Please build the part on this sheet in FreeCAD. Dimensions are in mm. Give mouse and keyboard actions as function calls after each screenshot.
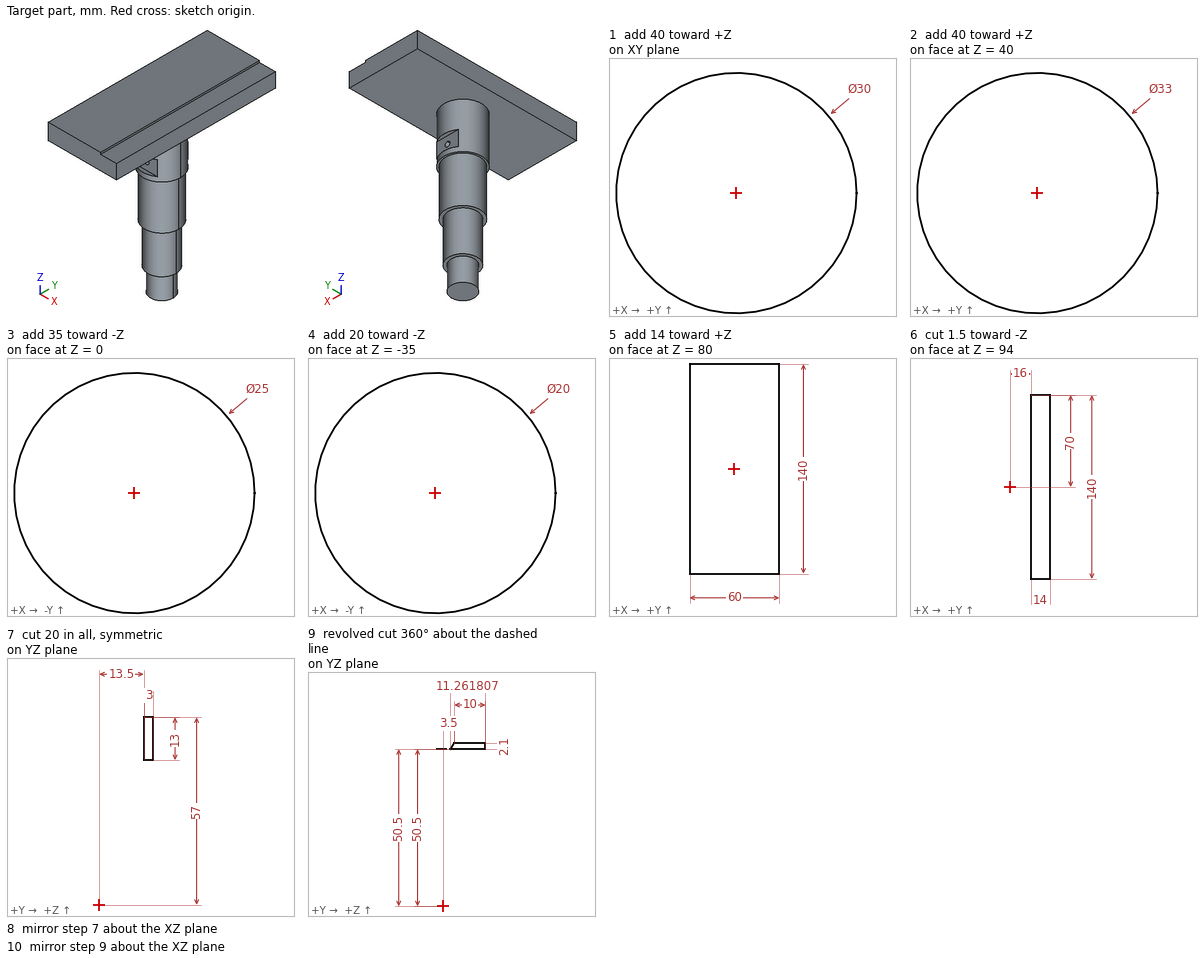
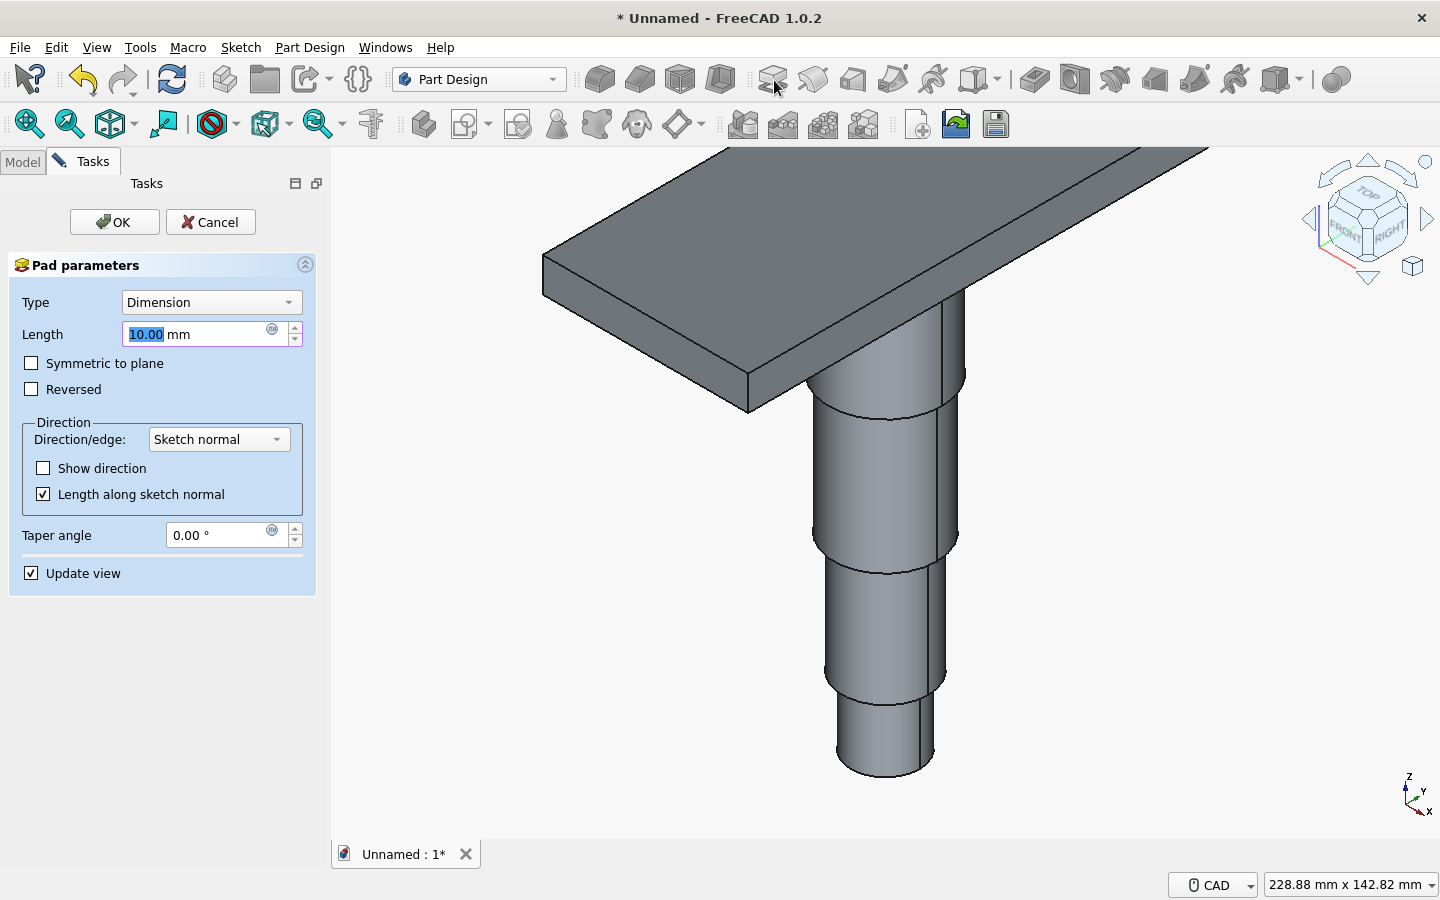
text(14)
key(Tab)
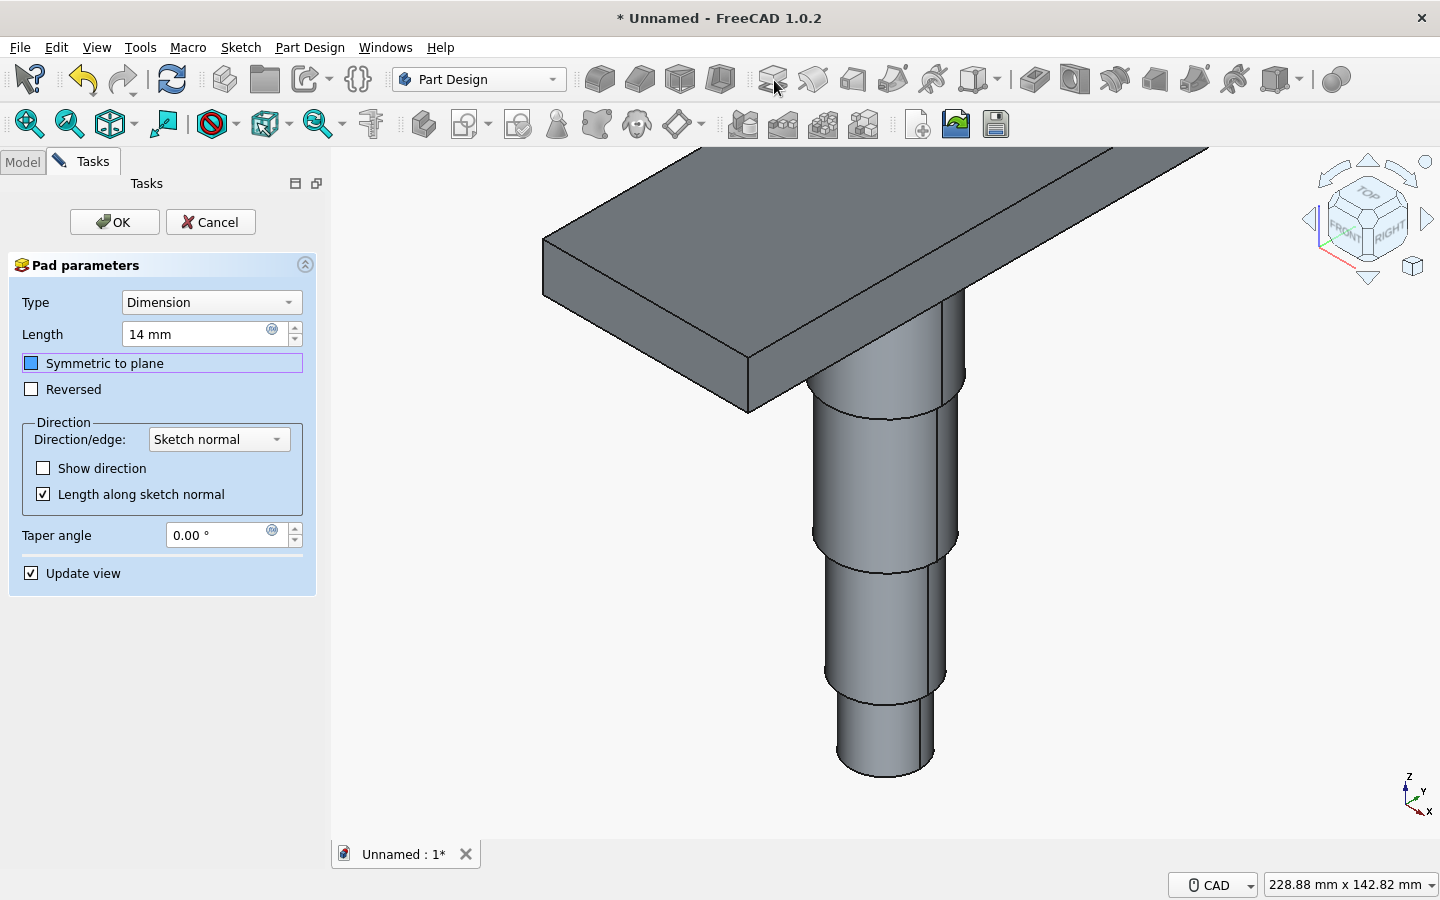
click(115, 222)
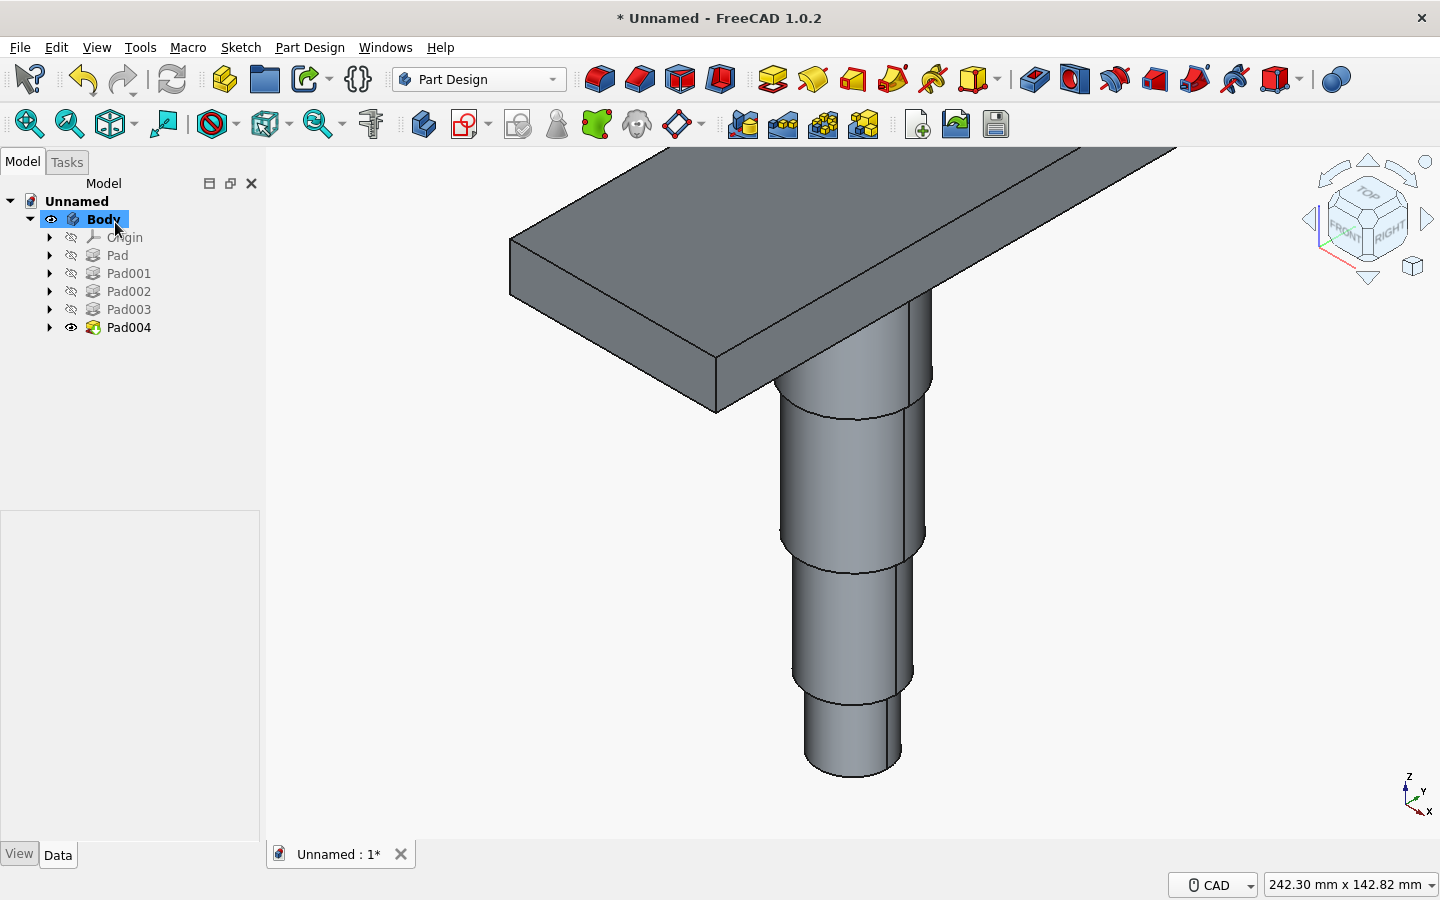
click(30, 124)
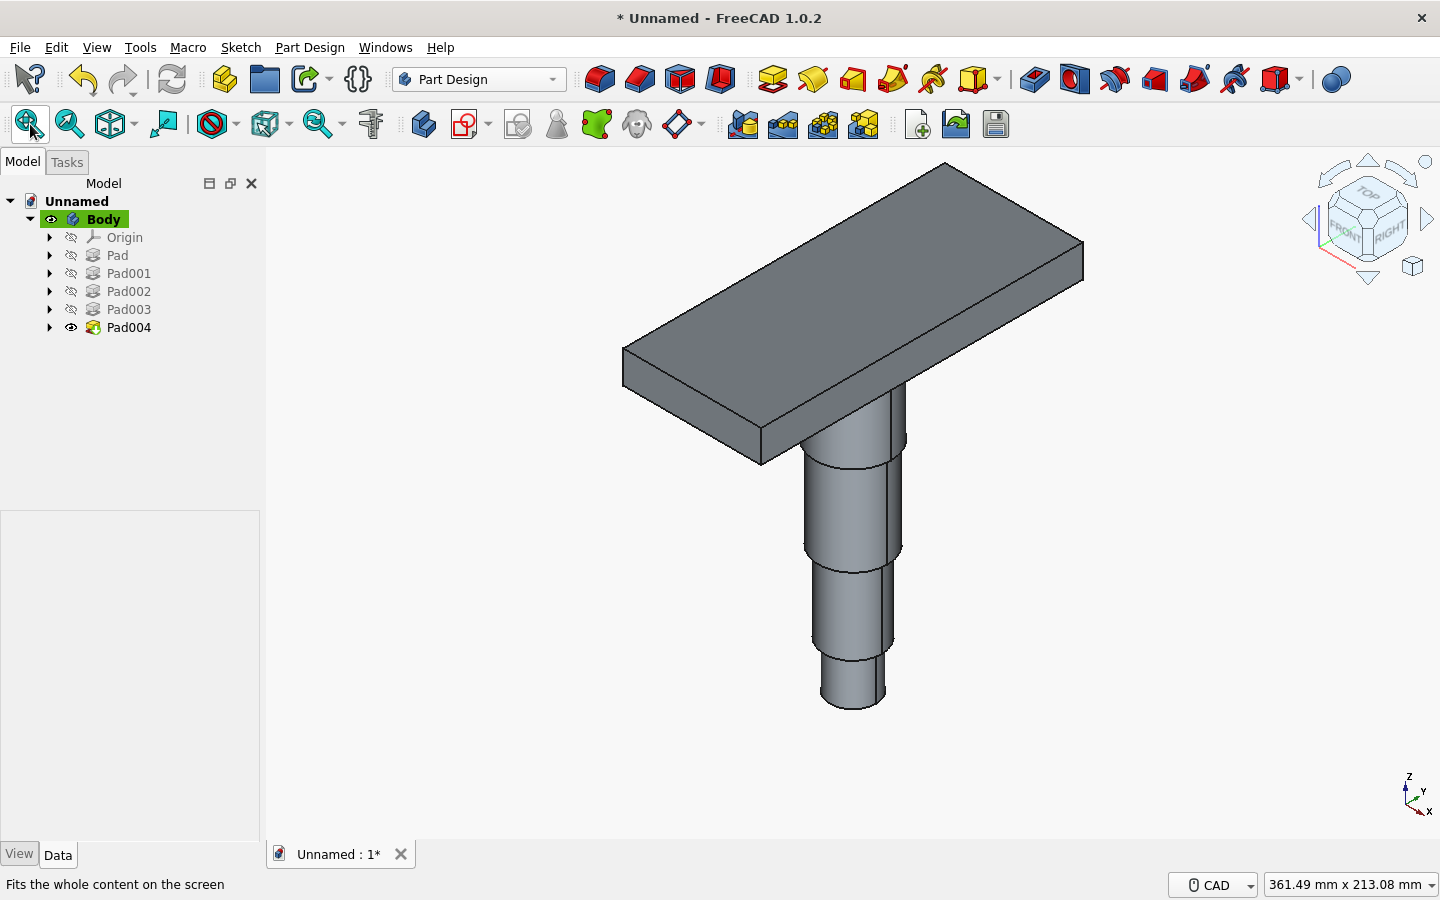
click(945, 241)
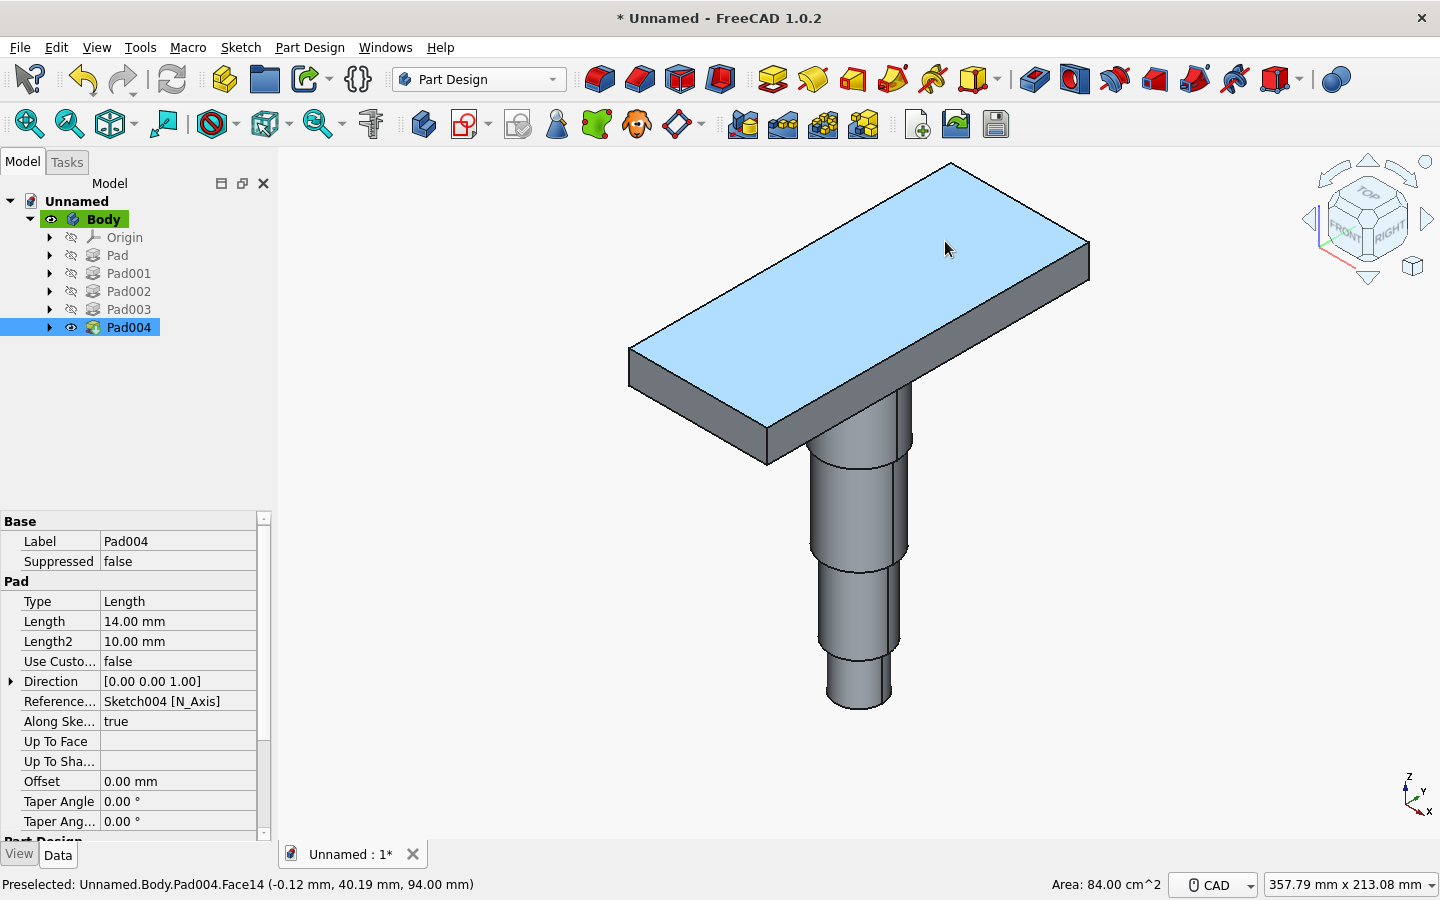
click(464, 124)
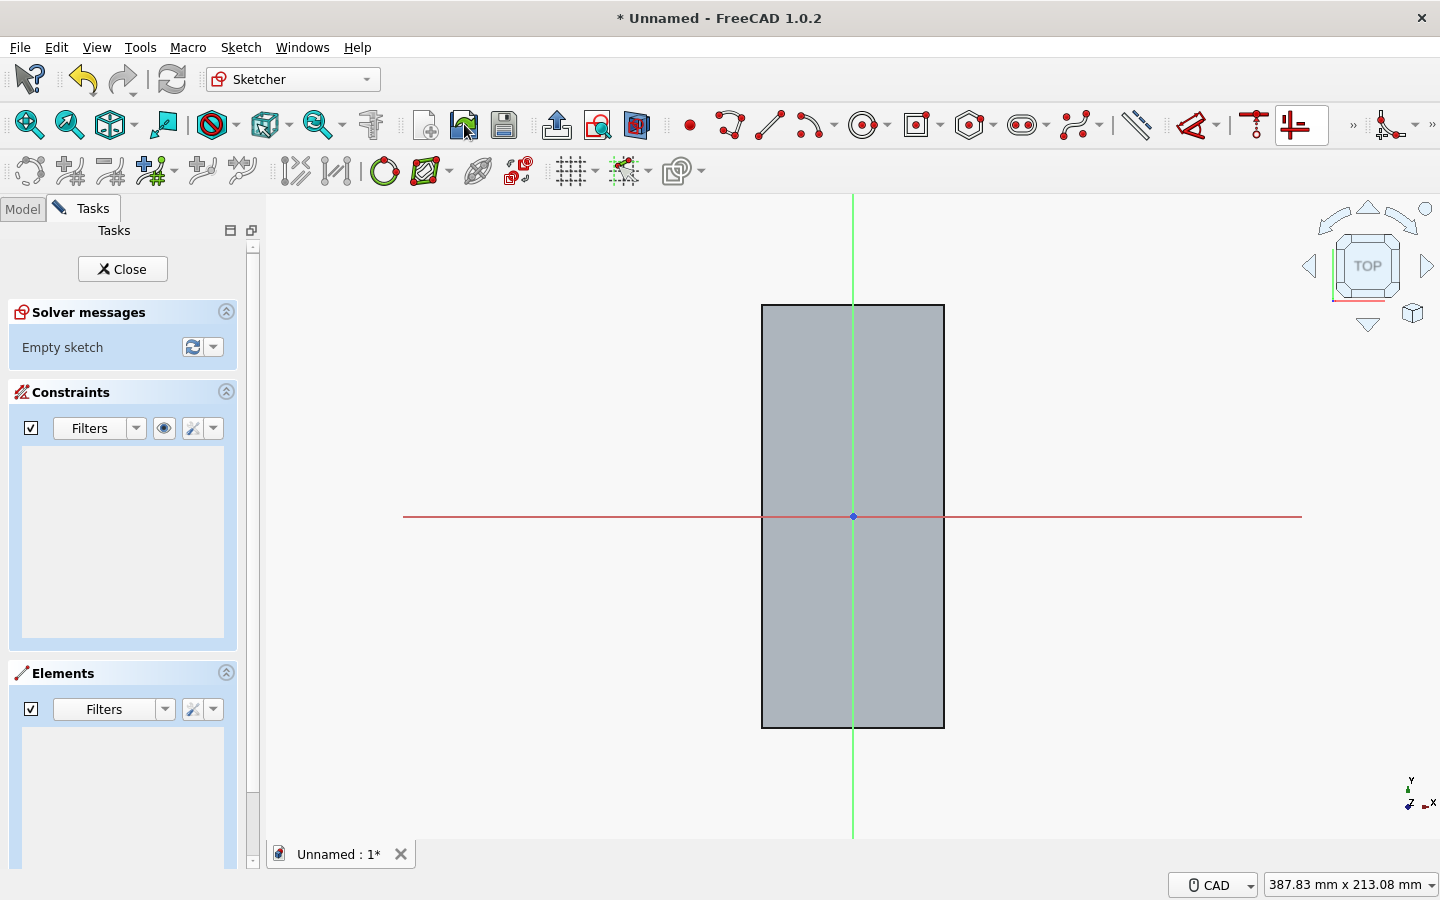
key(g)
key(r)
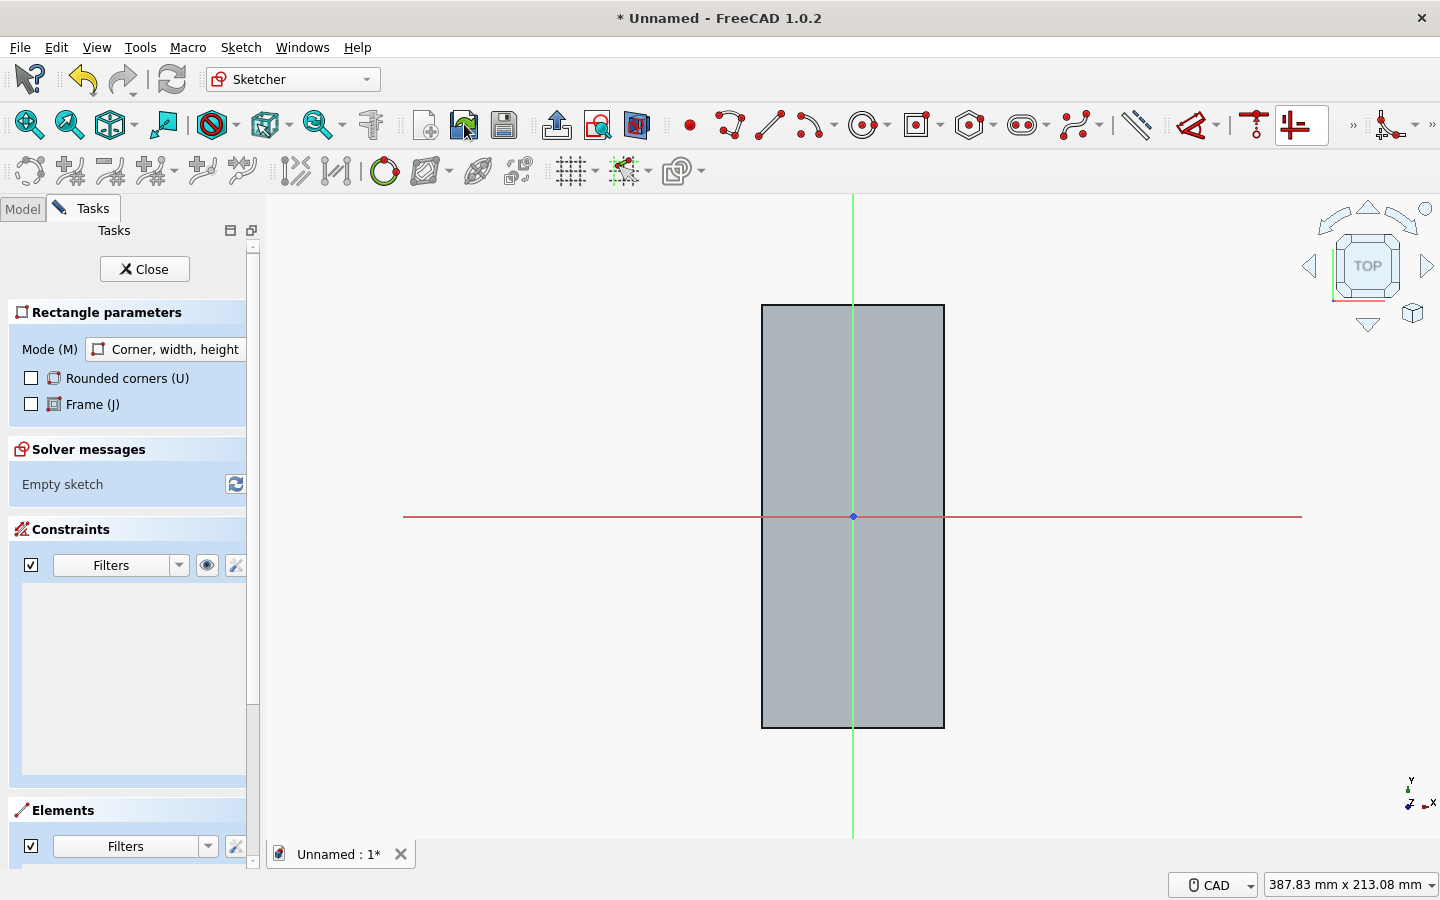
click(901, 305)
move(944, 728)